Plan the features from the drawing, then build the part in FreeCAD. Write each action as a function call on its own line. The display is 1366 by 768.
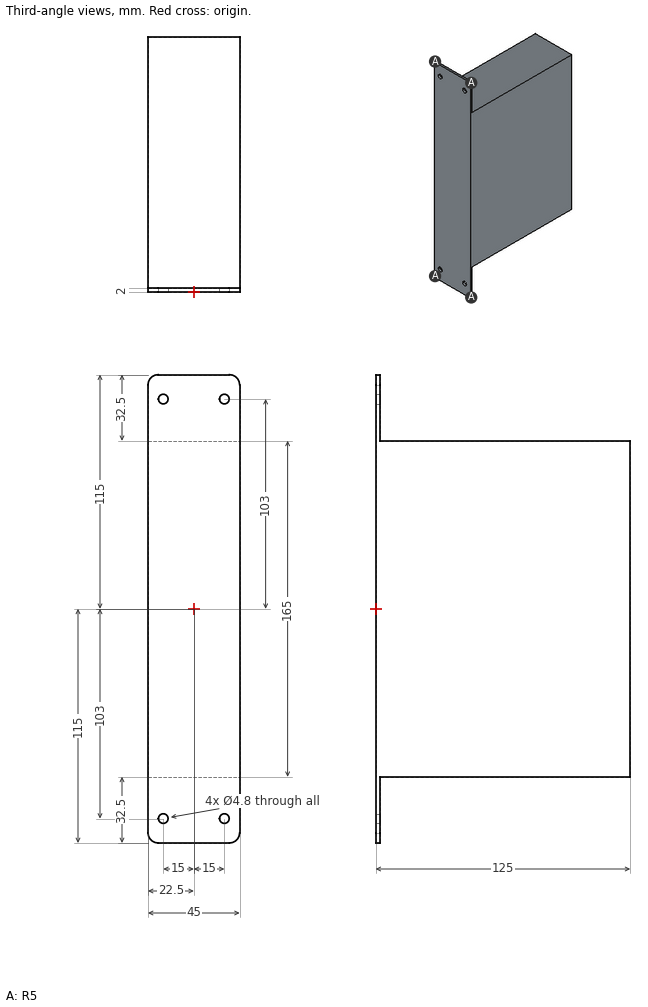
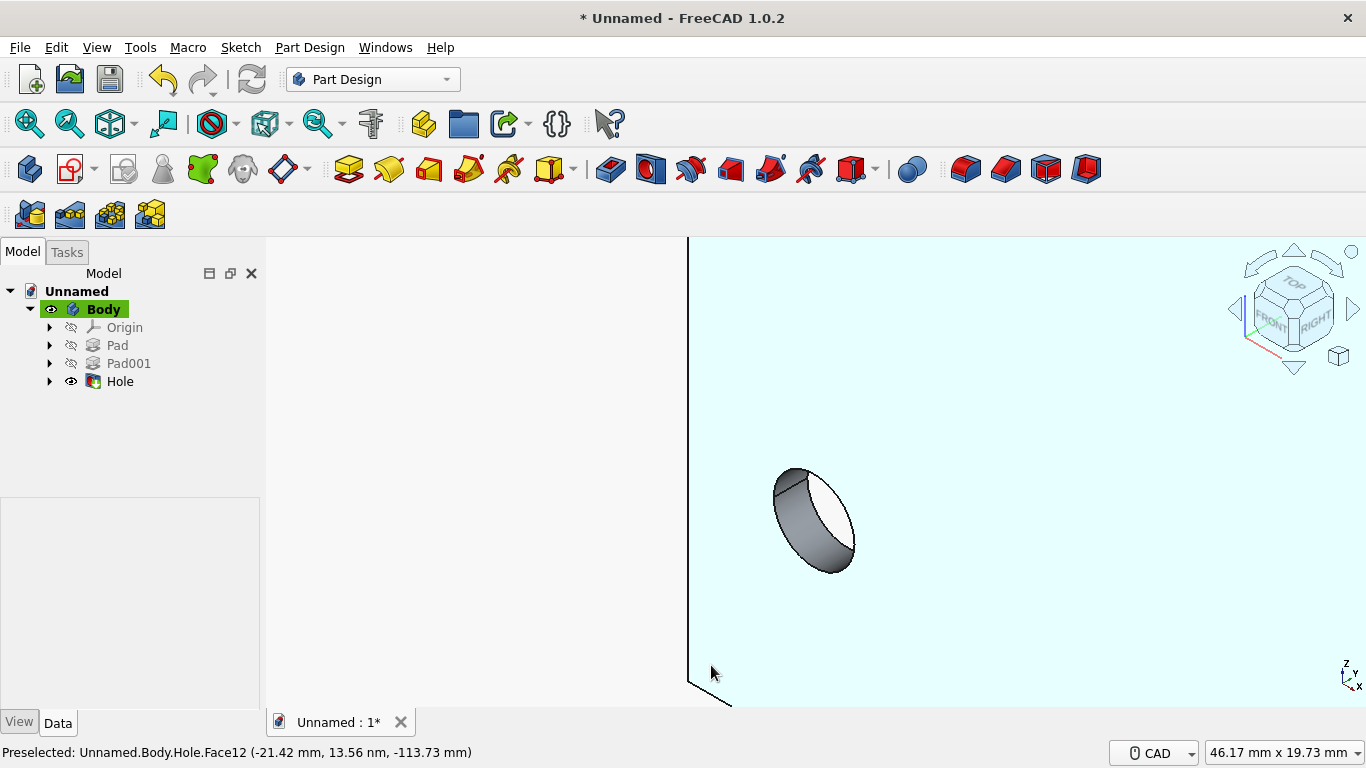
click(30, 124)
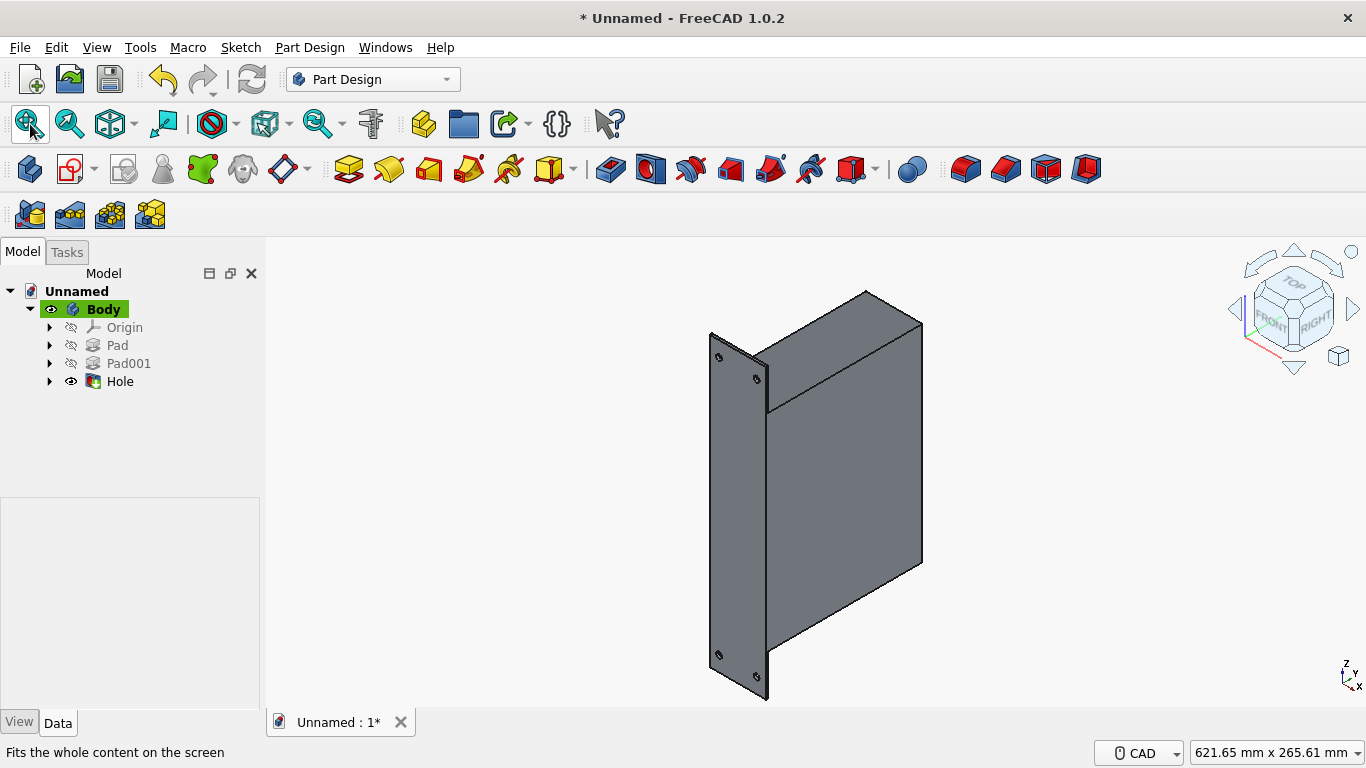
key(2)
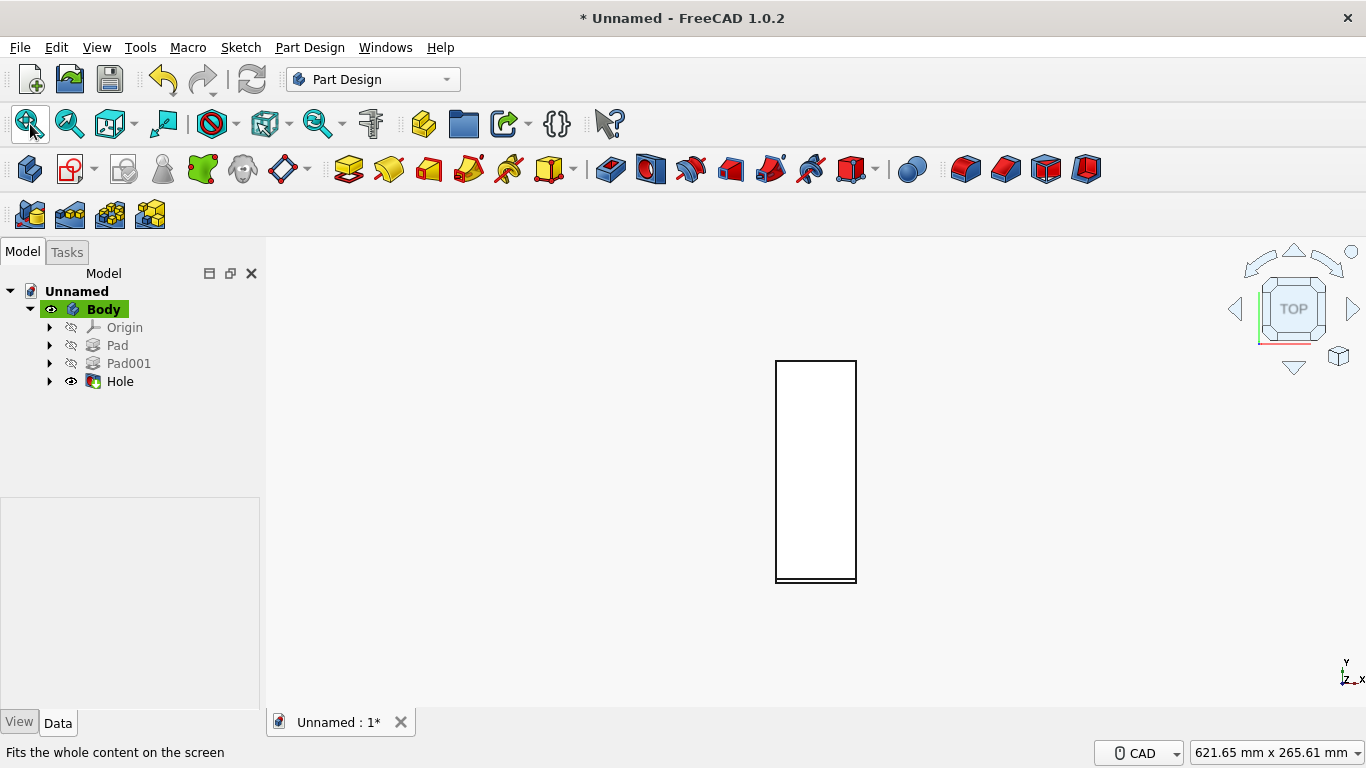
scroll(776, 580, up, 13)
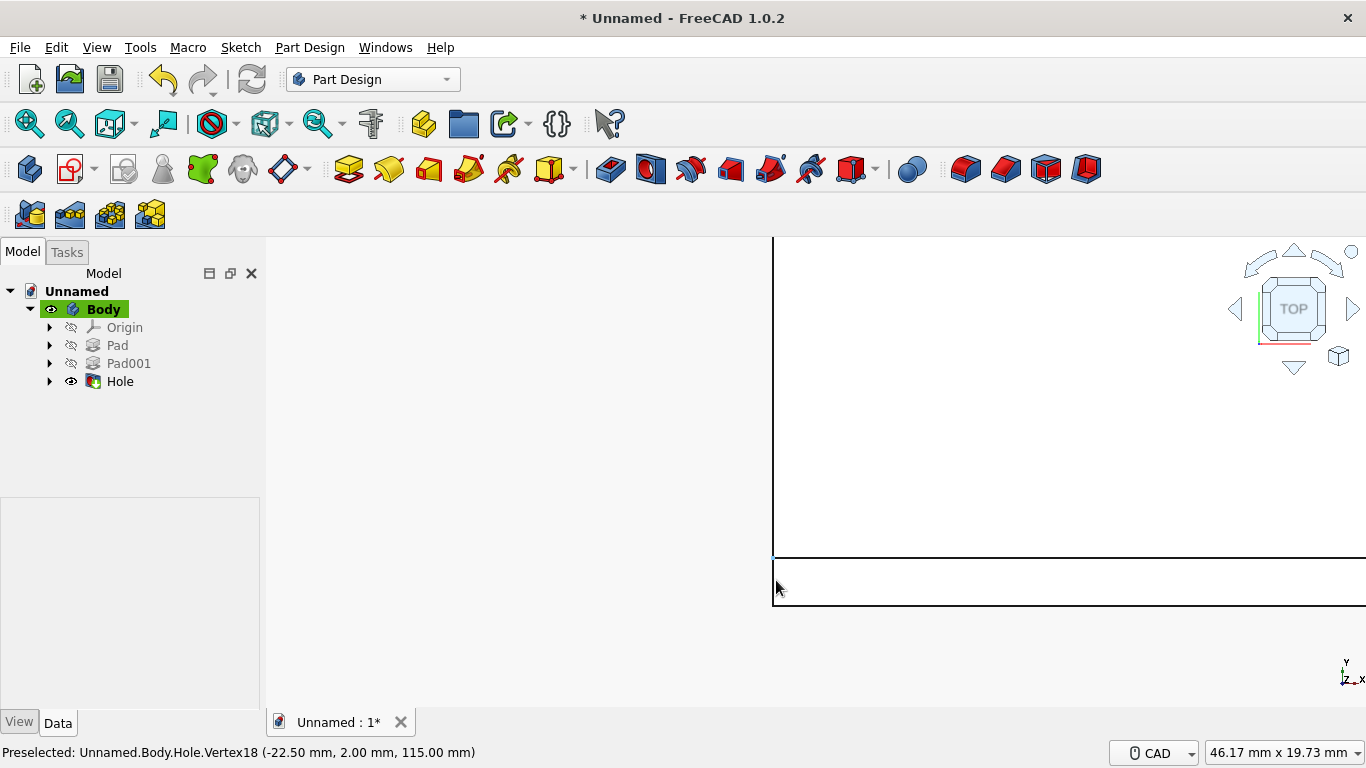
click(773, 581)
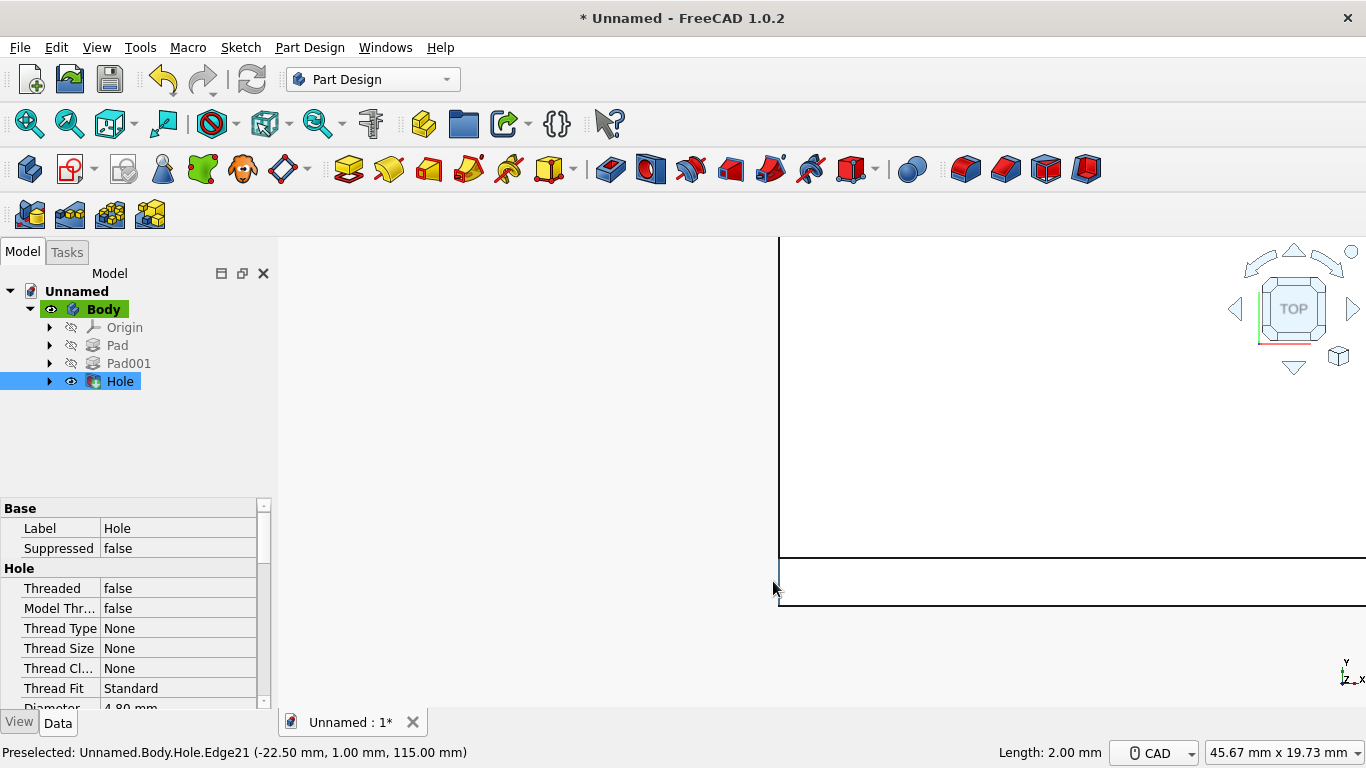
click(30, 124)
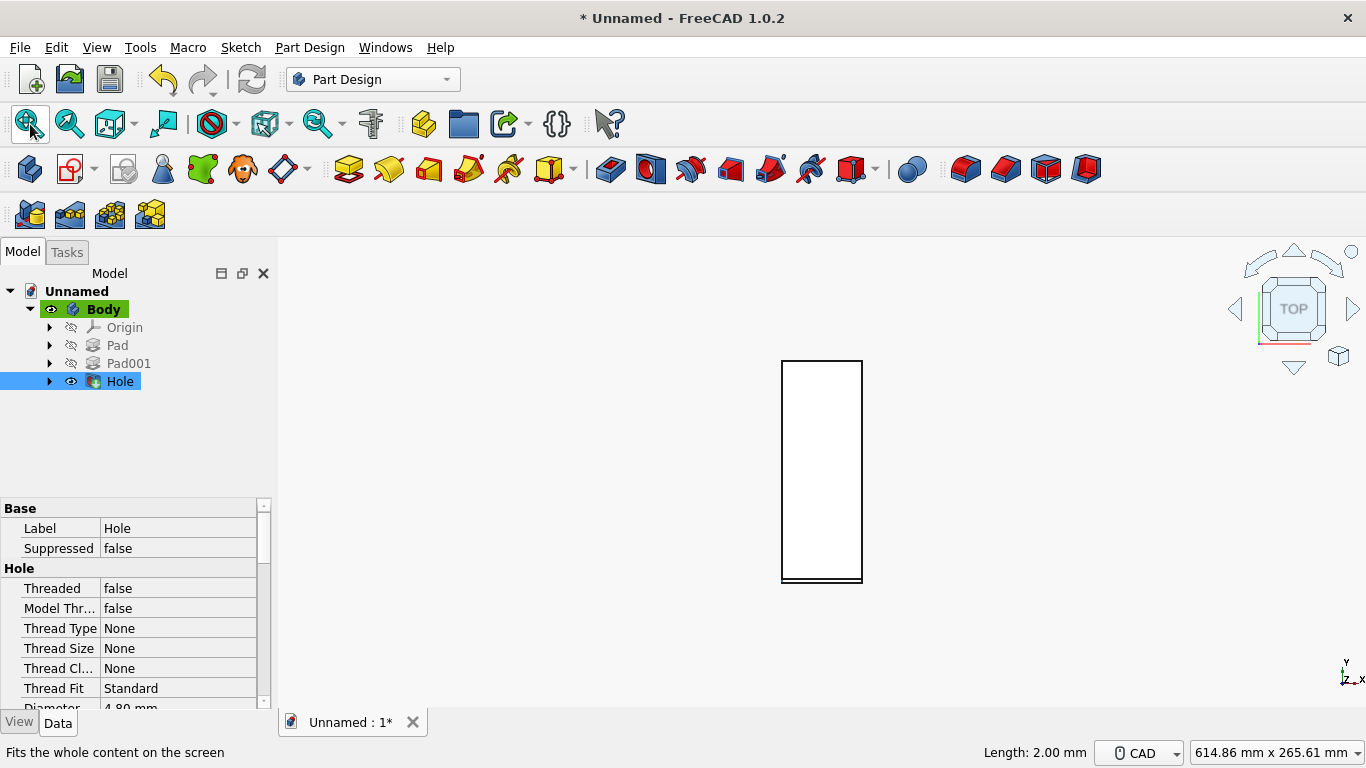
key(1)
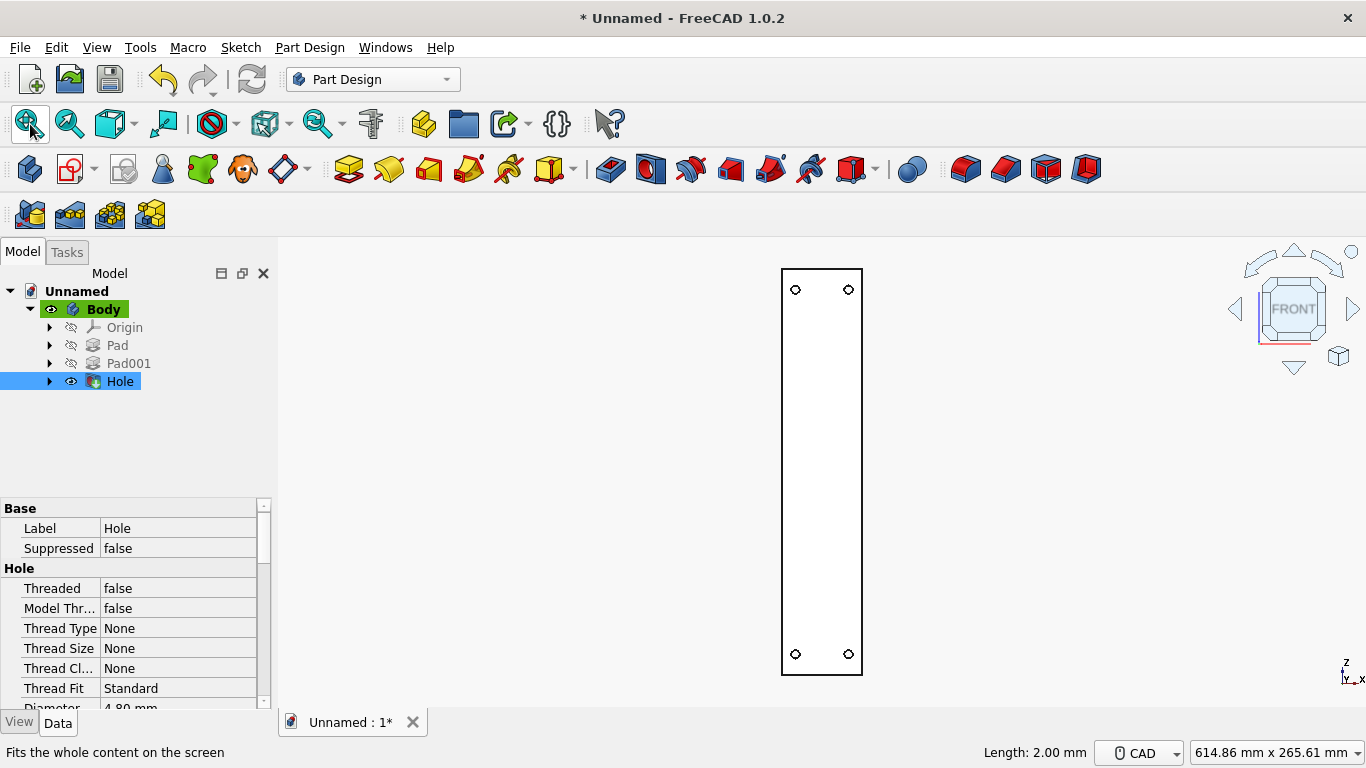
scroll(782, 674, up, 13)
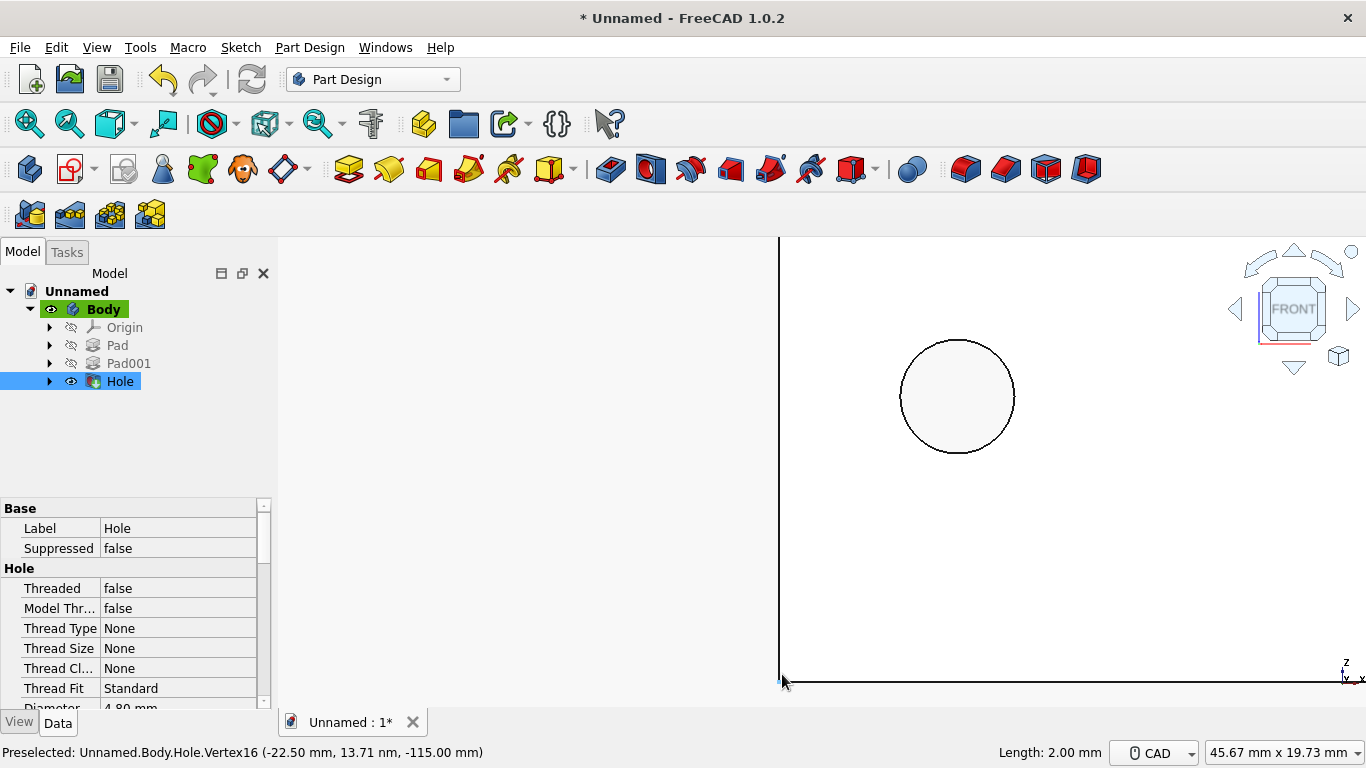
click(30, 124)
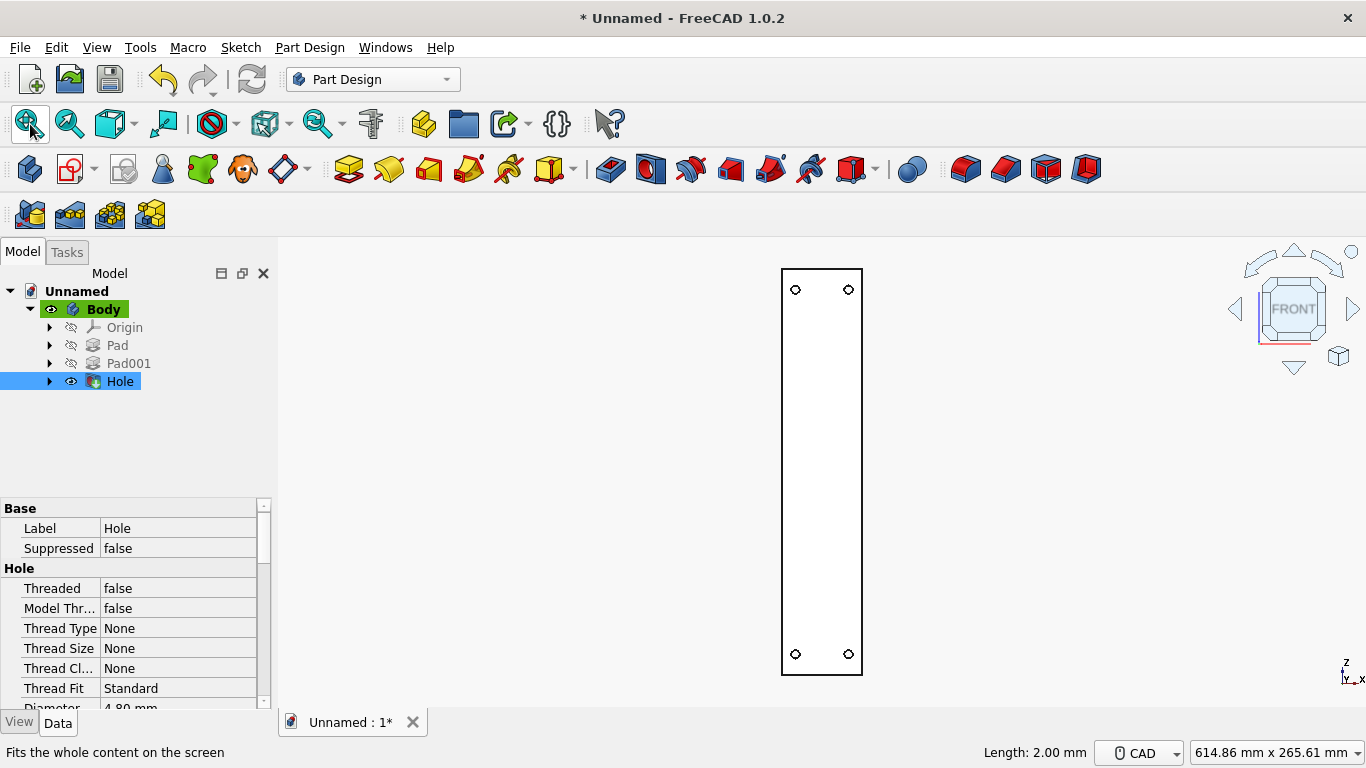
key(3)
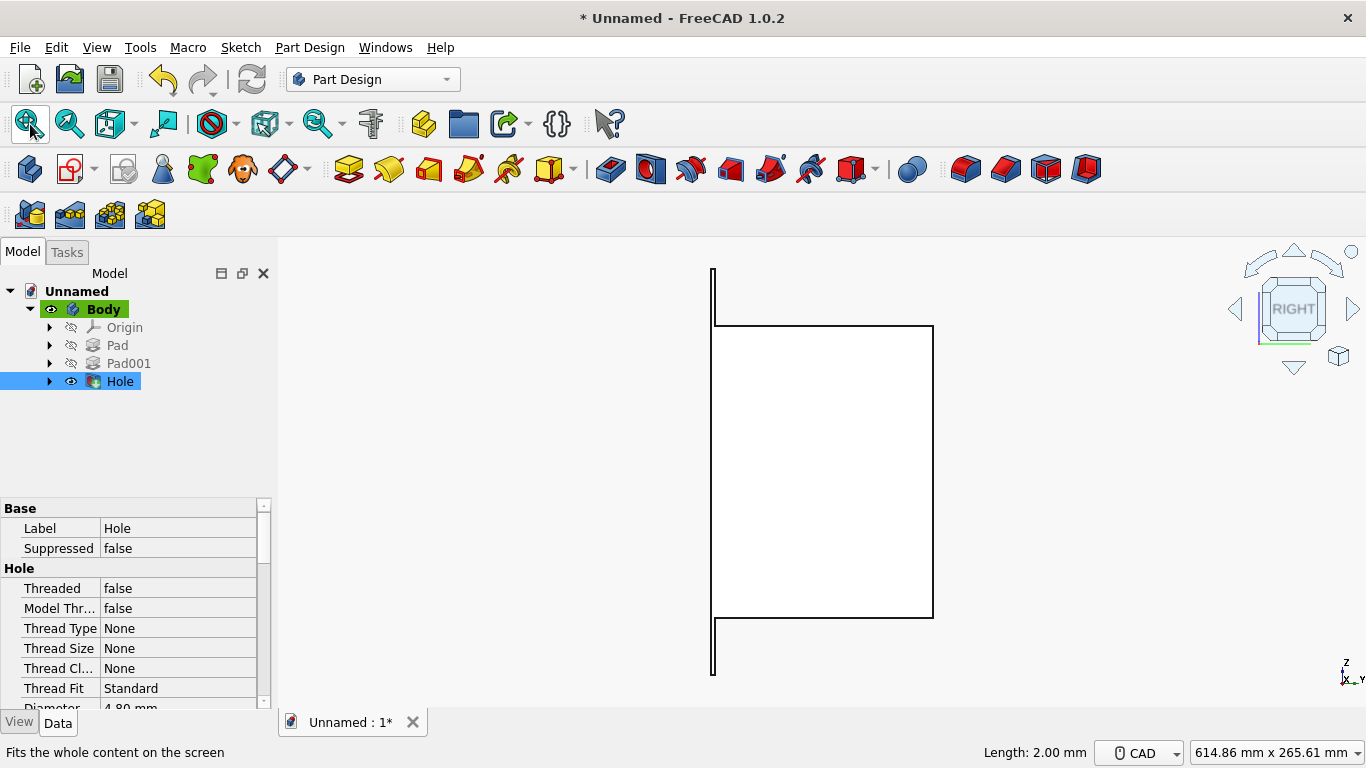
scroll(713, 674, up, 13)